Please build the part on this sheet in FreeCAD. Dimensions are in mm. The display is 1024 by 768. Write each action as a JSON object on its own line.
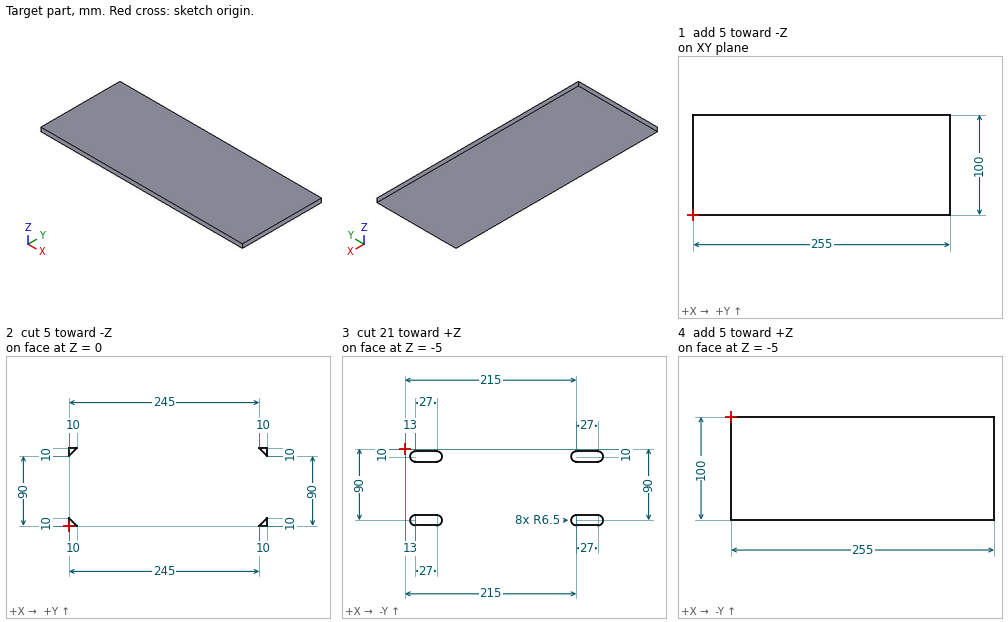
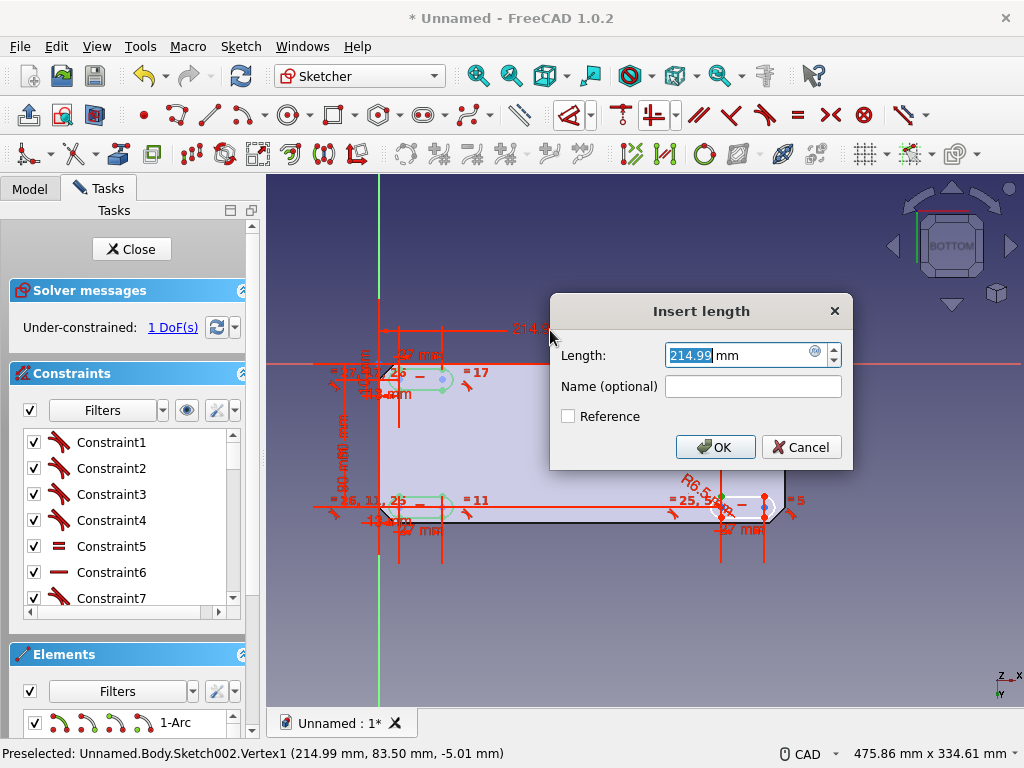
{"action": "type", "text": "215"}
{"action": "key", "text": "Return"}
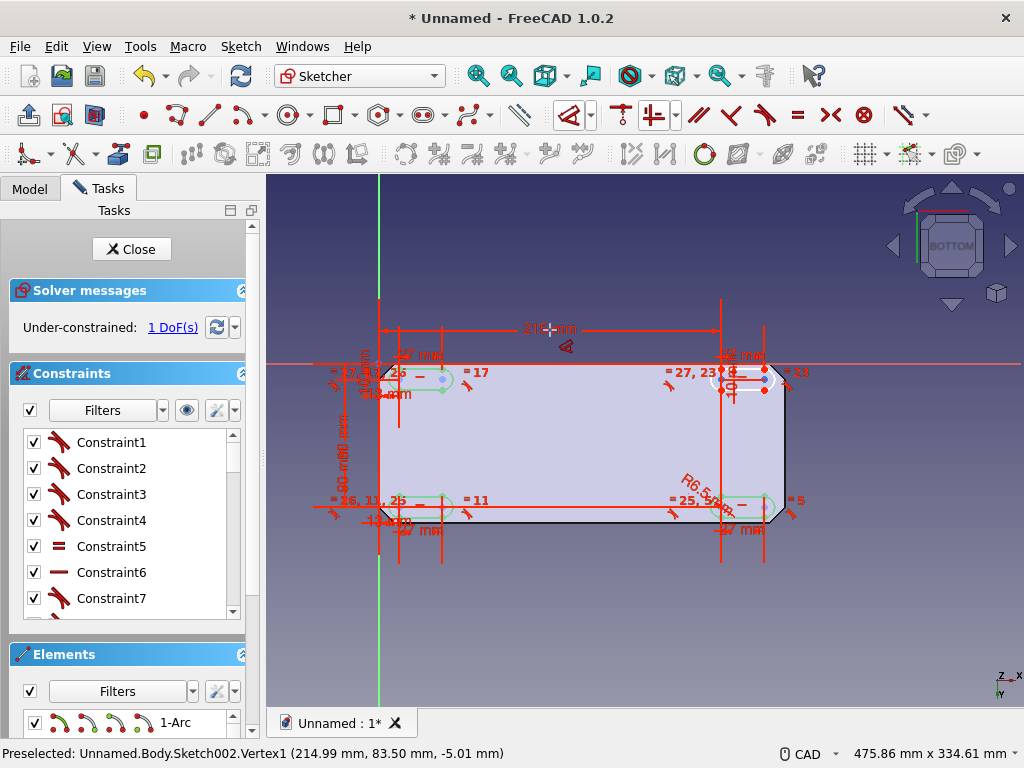
{"action": "left_click", "coordinate": [721, 369]}
{"action": "left_click", "coordinate": [471, 330]}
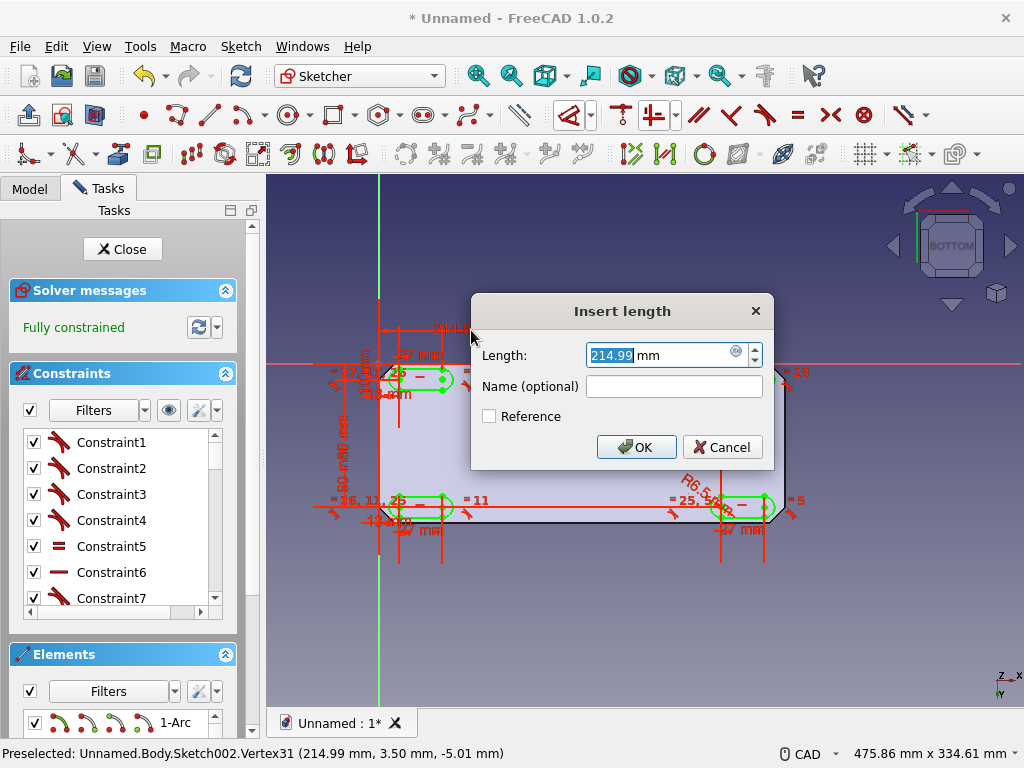
{"action": "type", "text": "215"}
{"action": "key", "text": "Return"}
{"action": "key", "text": "Escape"}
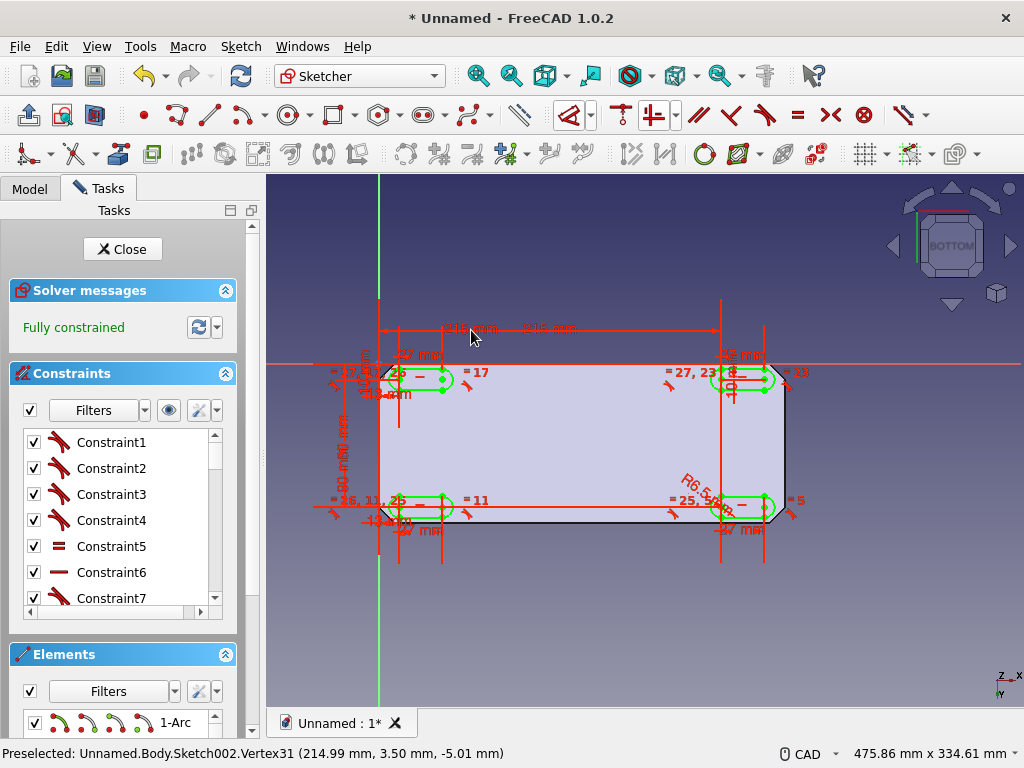
{"action": "left_click", "coordinate": [123, 249]}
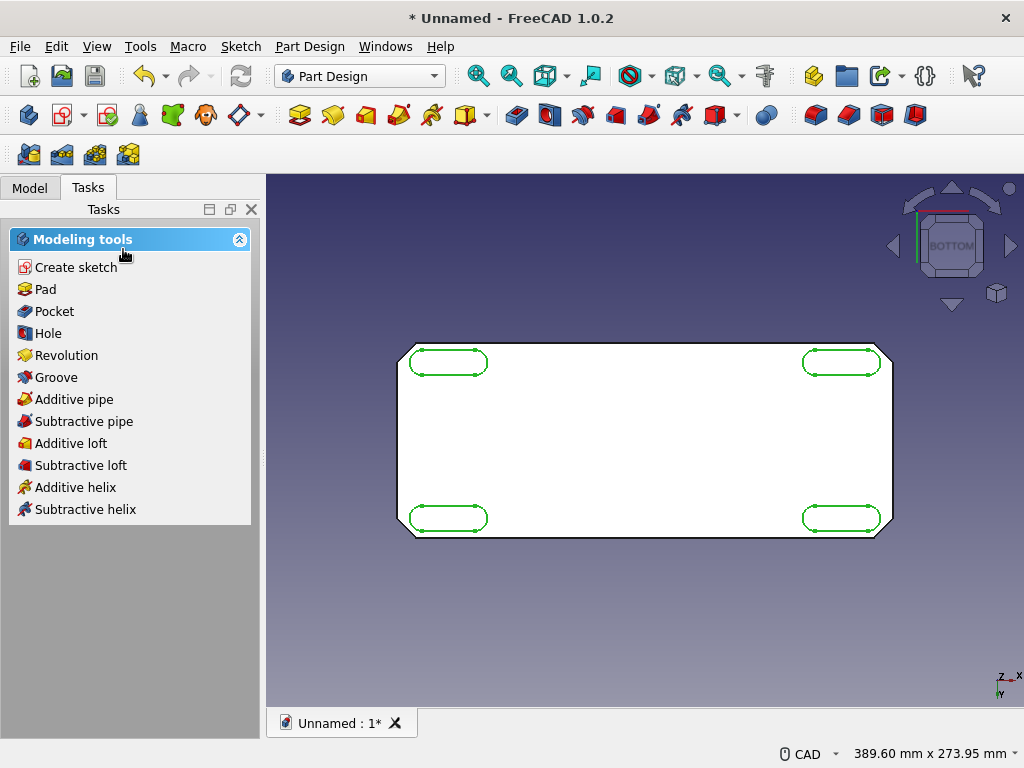
{"action": "left_click", "coordinate": [517, 116]}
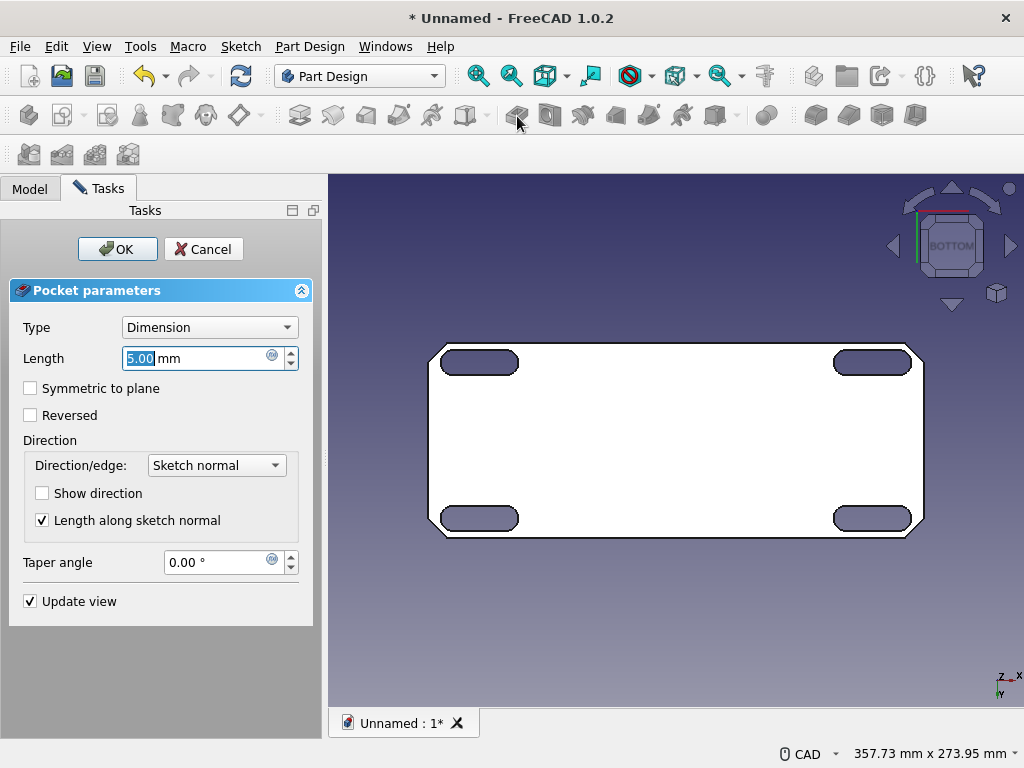
{"action": "type", "text": "21"}
{"action": "key", "text": "Tab"}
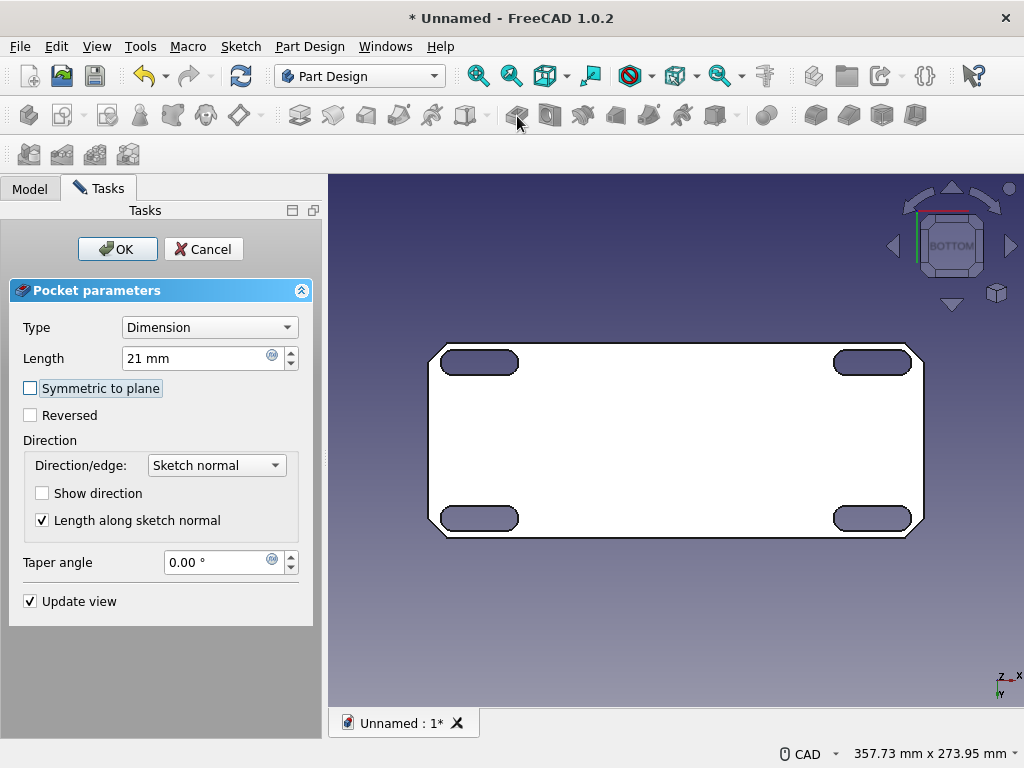
{"action": "left_click", "coordinate": [118, 249]}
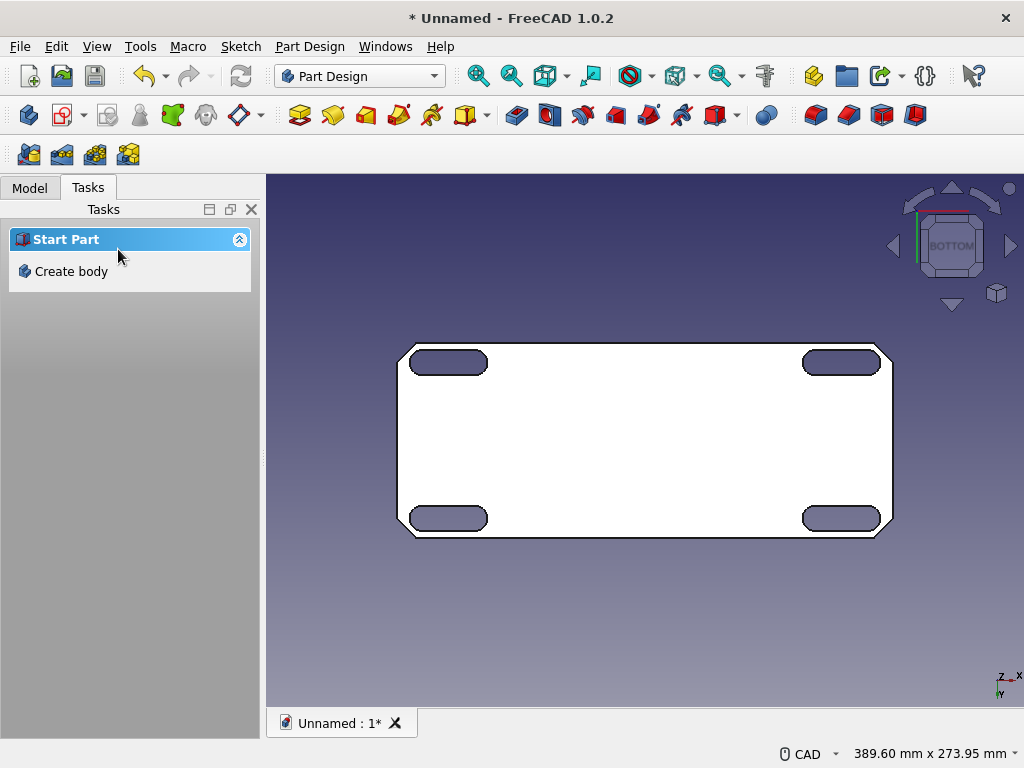
{"action": "left_click", "coordinate": [716, 440]}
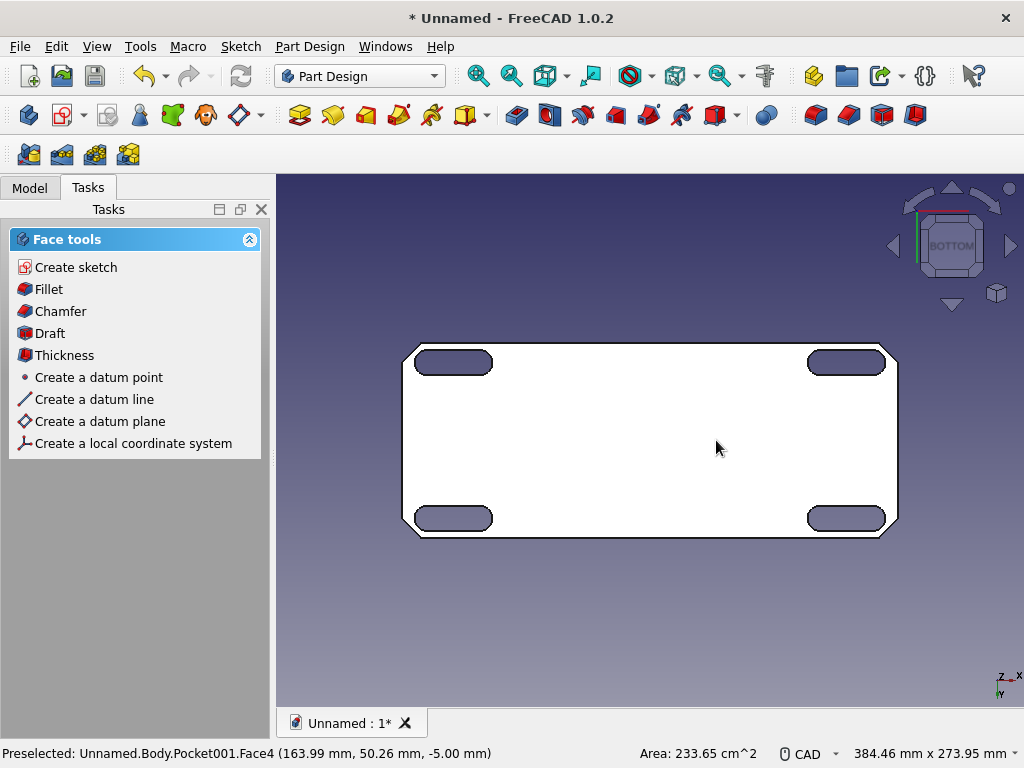
{"action": "left_click", "coordinate": [62, 116]}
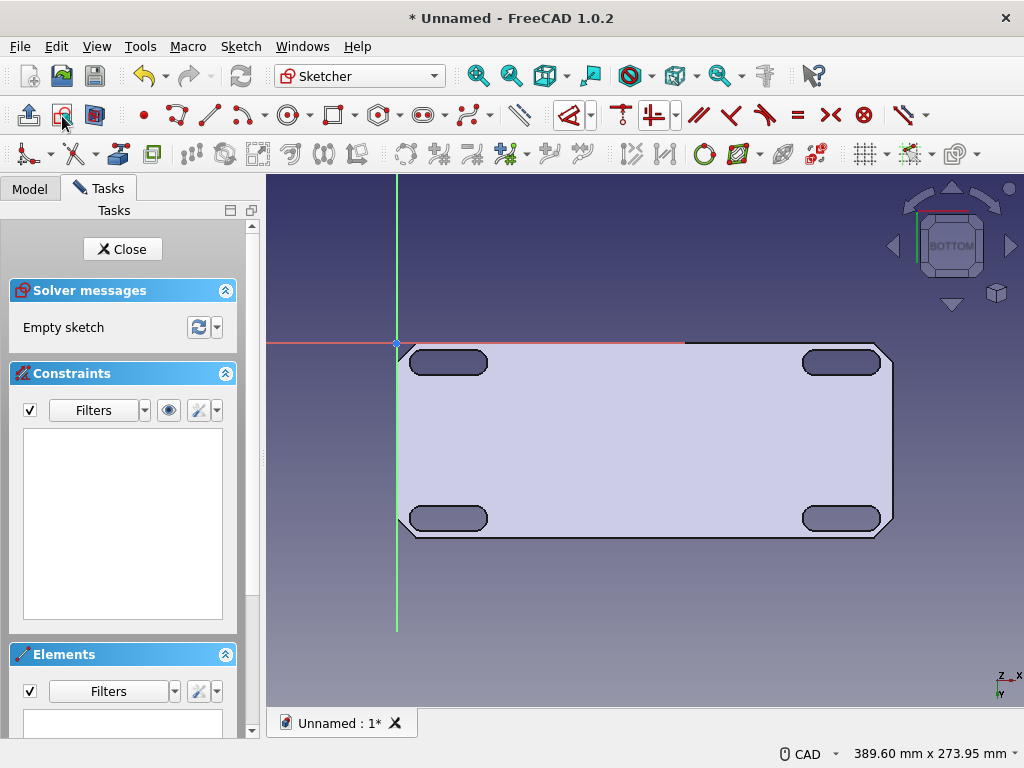
{"action": "scroll", "coordinate": [294, 440], "scroll_direction": "down", "scroll_amount": 1}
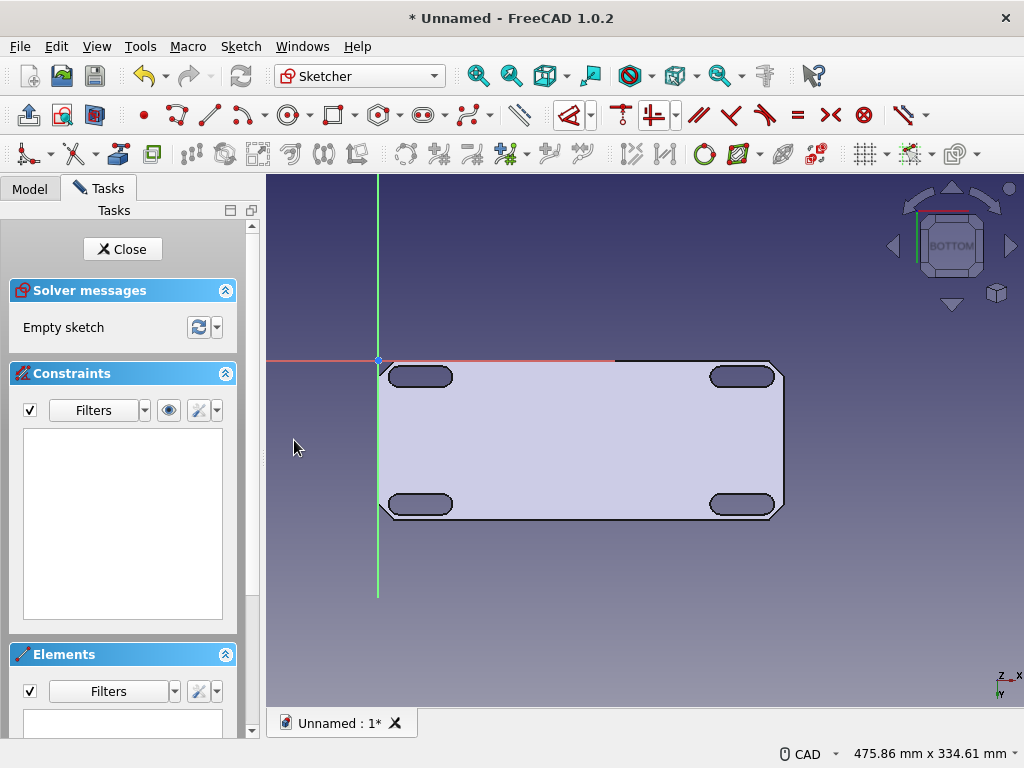
{"action": "key", "text": "g r"}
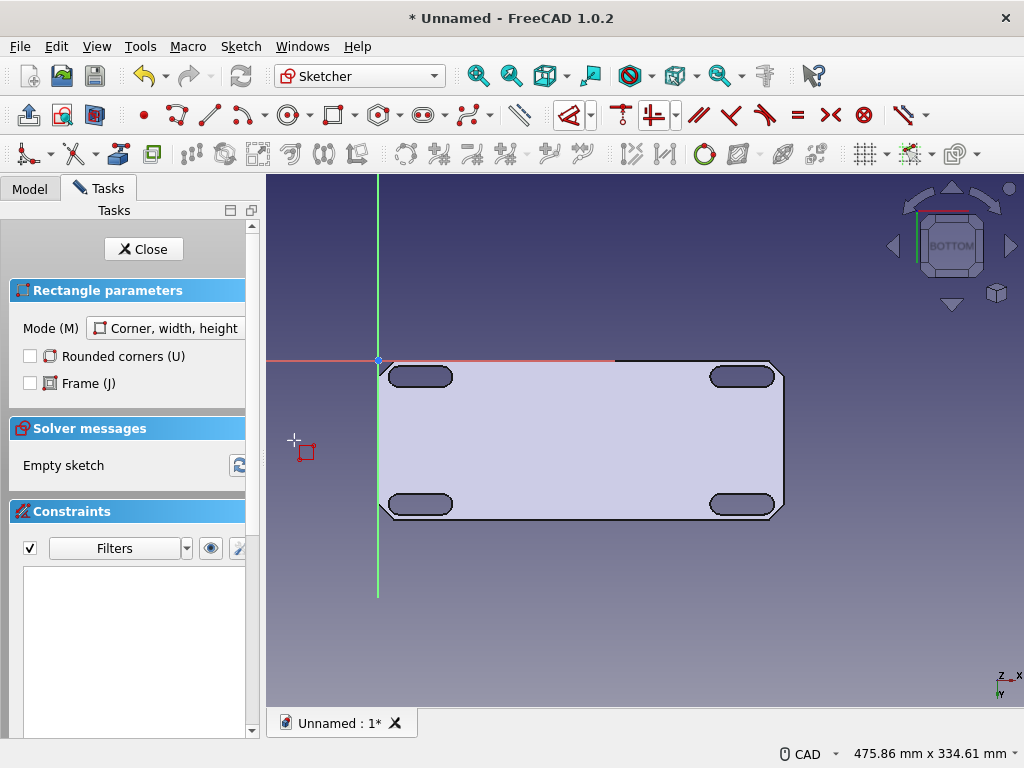
{"action": "left_click", "coordinate": [378, 361]}
{"action": "left_click", "coordinate": [784, 520]}
{"action": "key", "text": "Escape"}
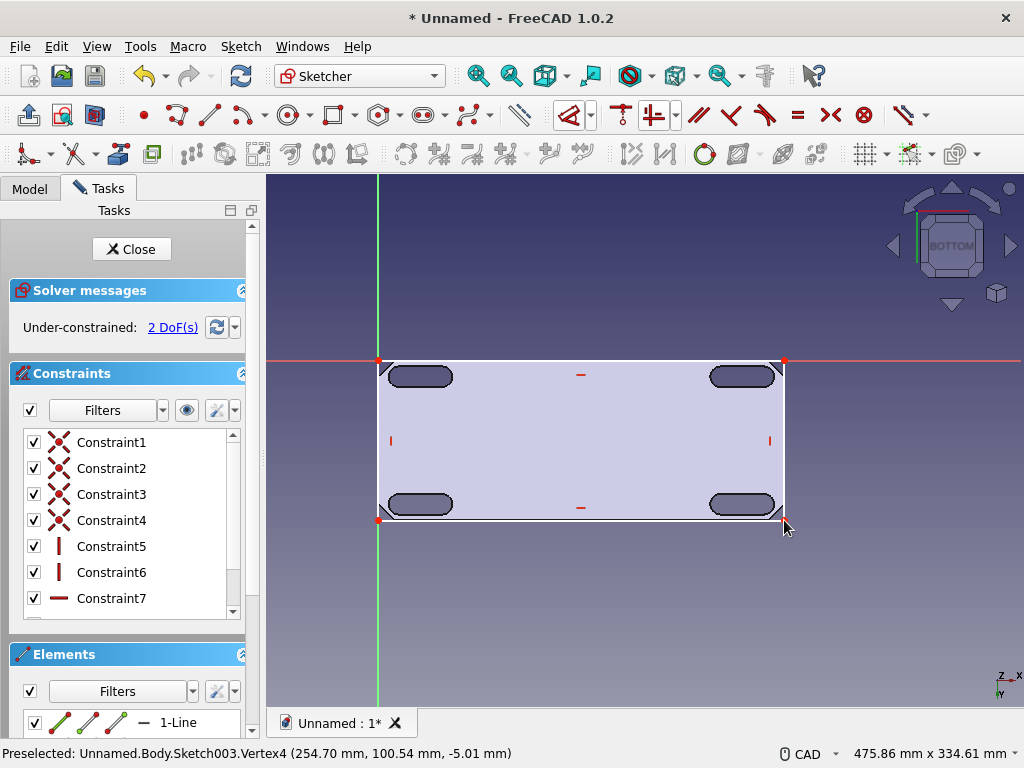
{"action": "key", "text": "d"}